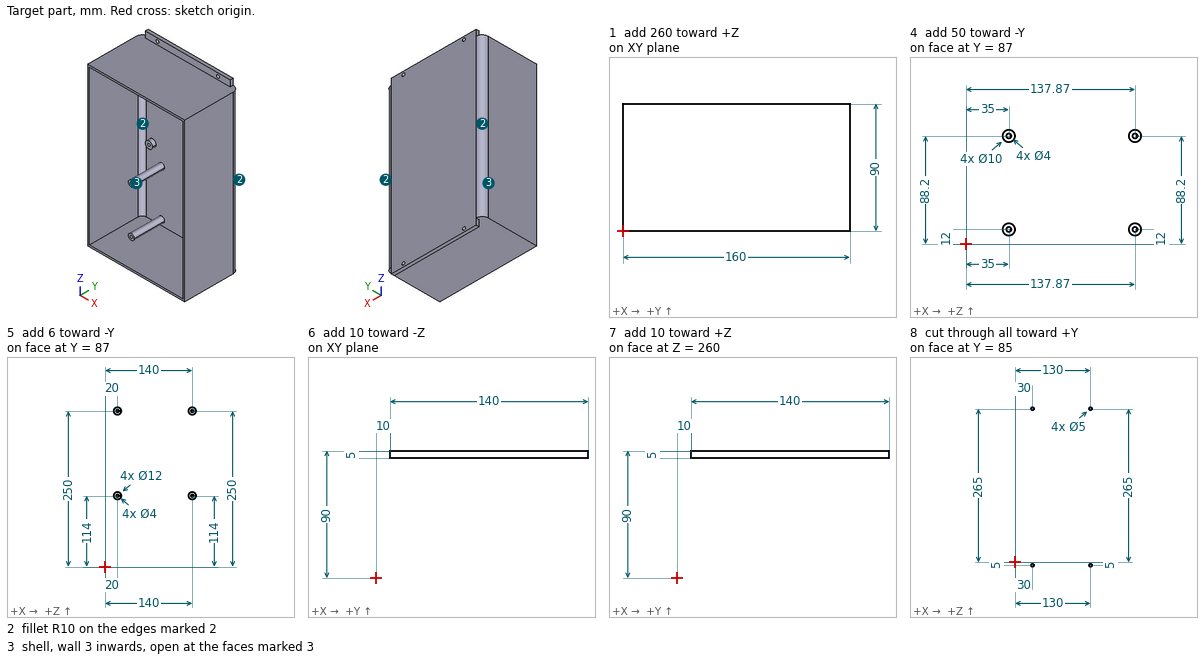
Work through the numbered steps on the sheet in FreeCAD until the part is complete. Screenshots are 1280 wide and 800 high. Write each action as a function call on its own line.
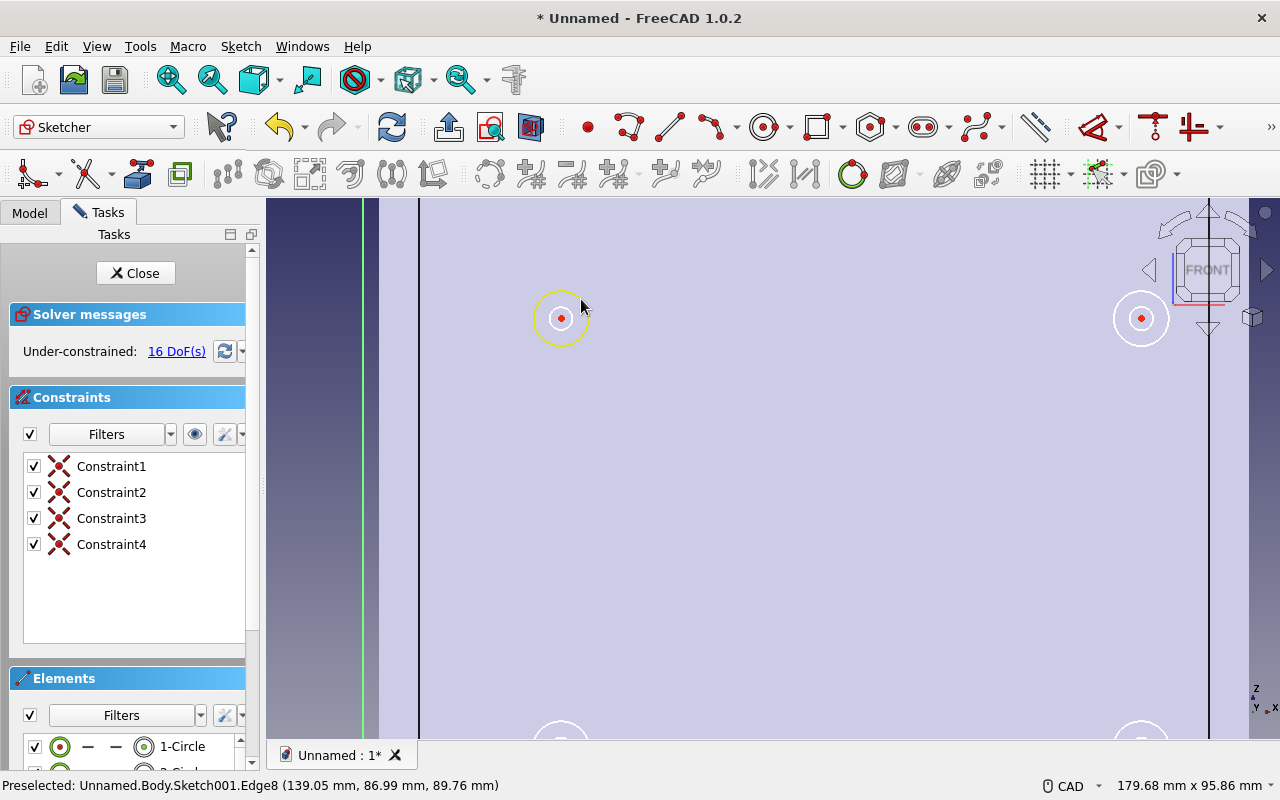
click(580, 299)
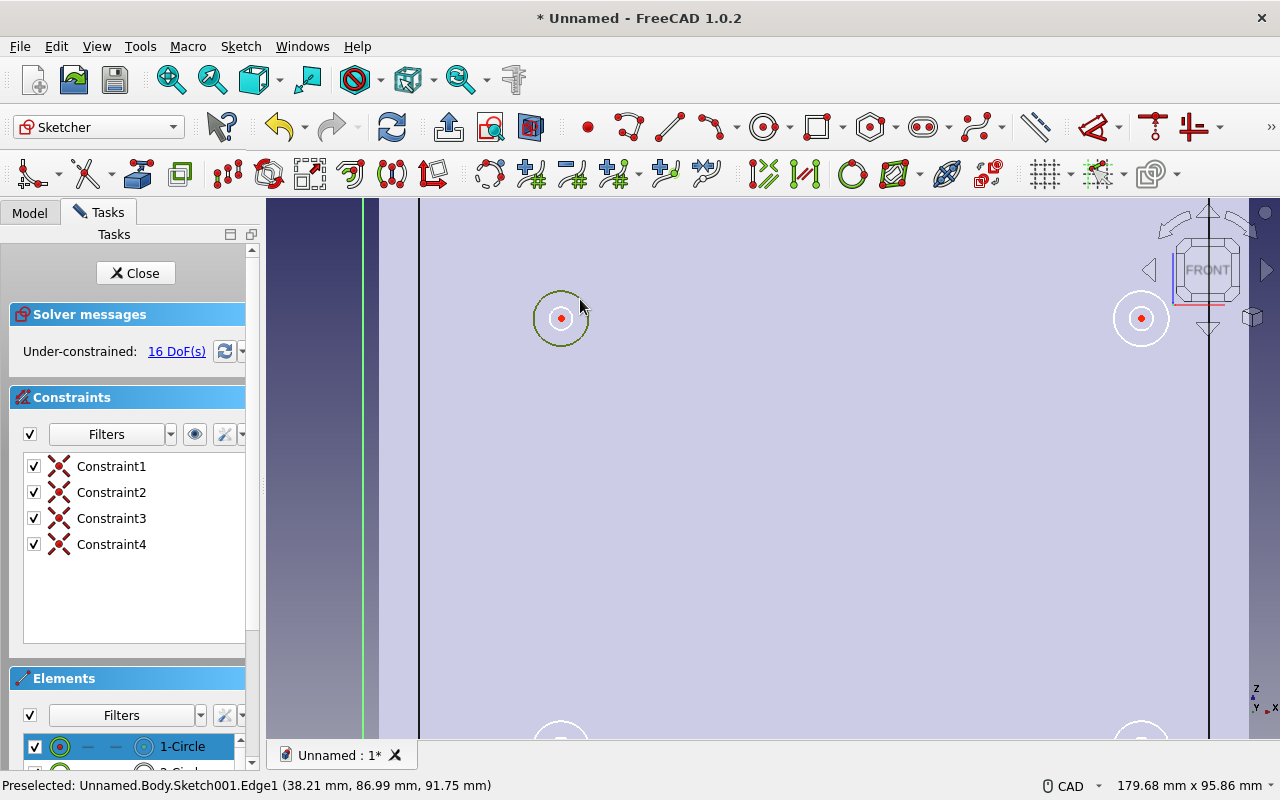
scroll(579, 298, down, 2)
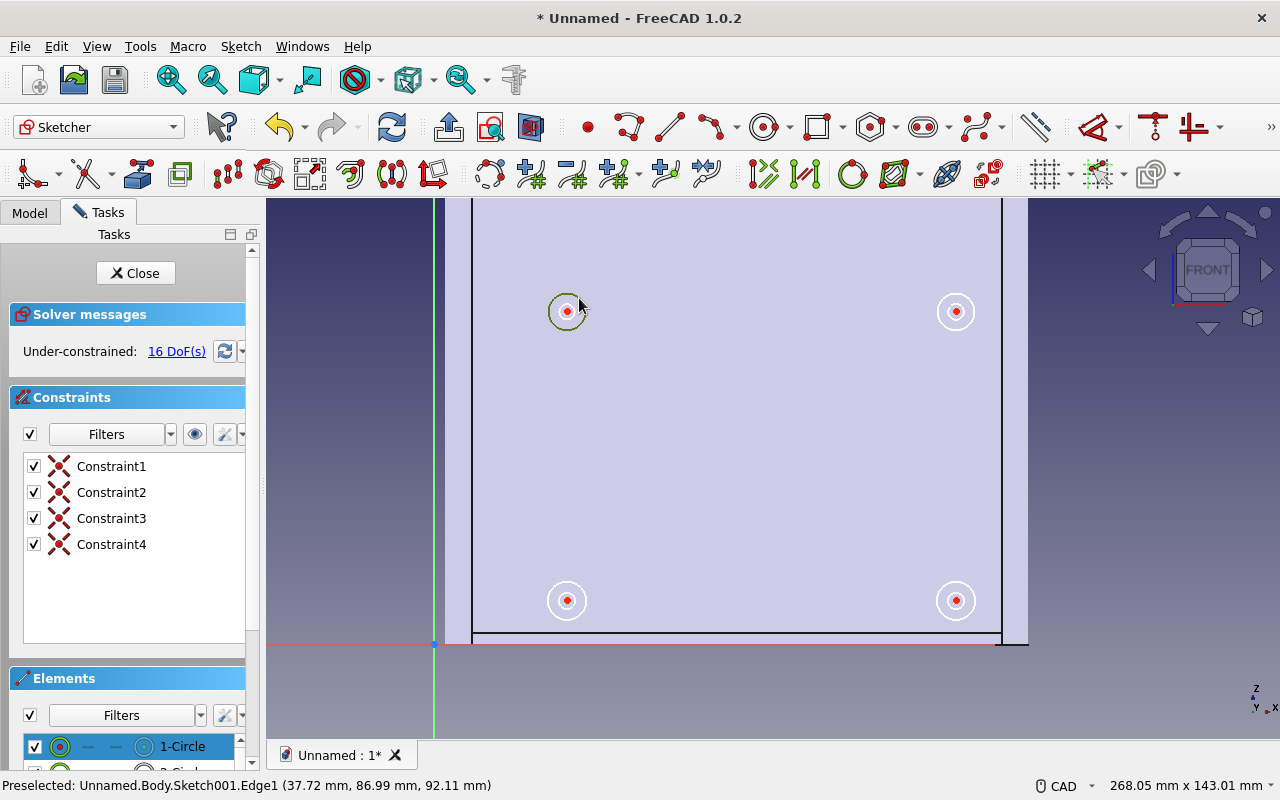
scroll(581, 587, up, 2)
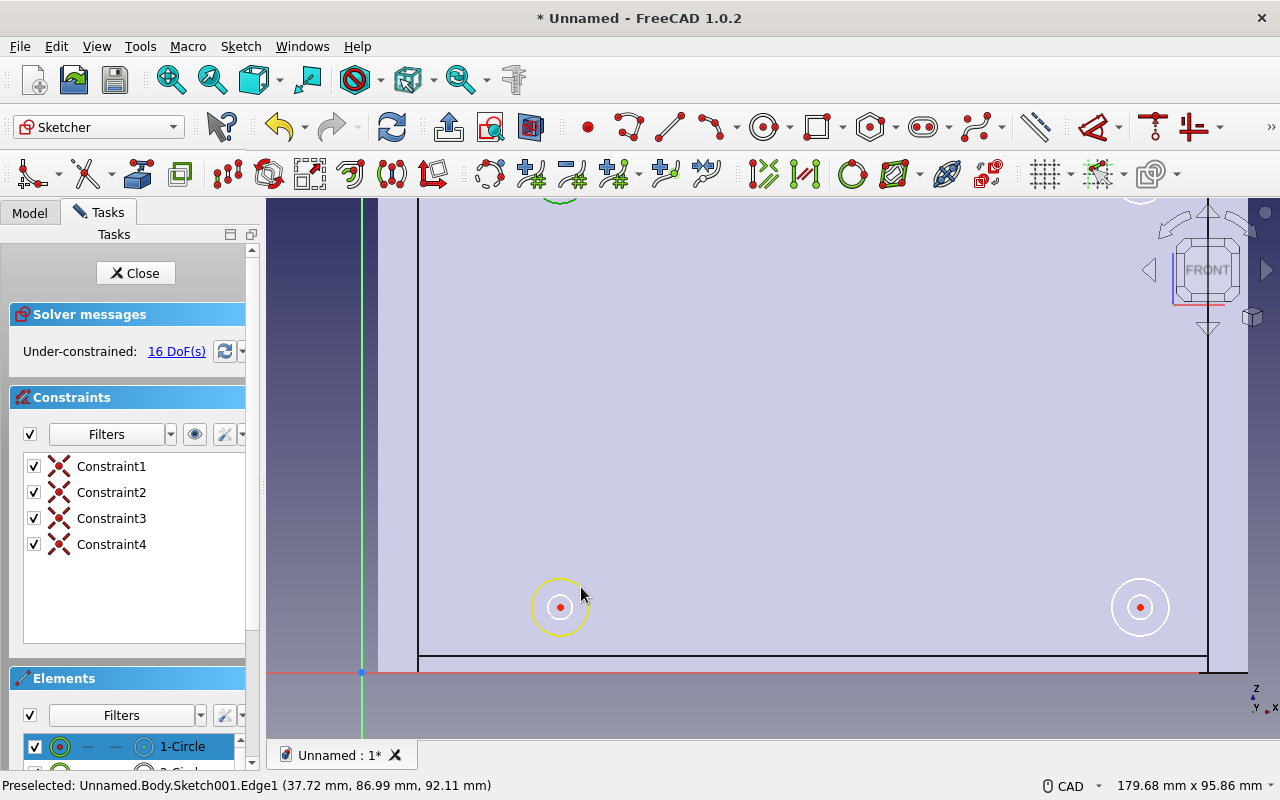
click(580, 587)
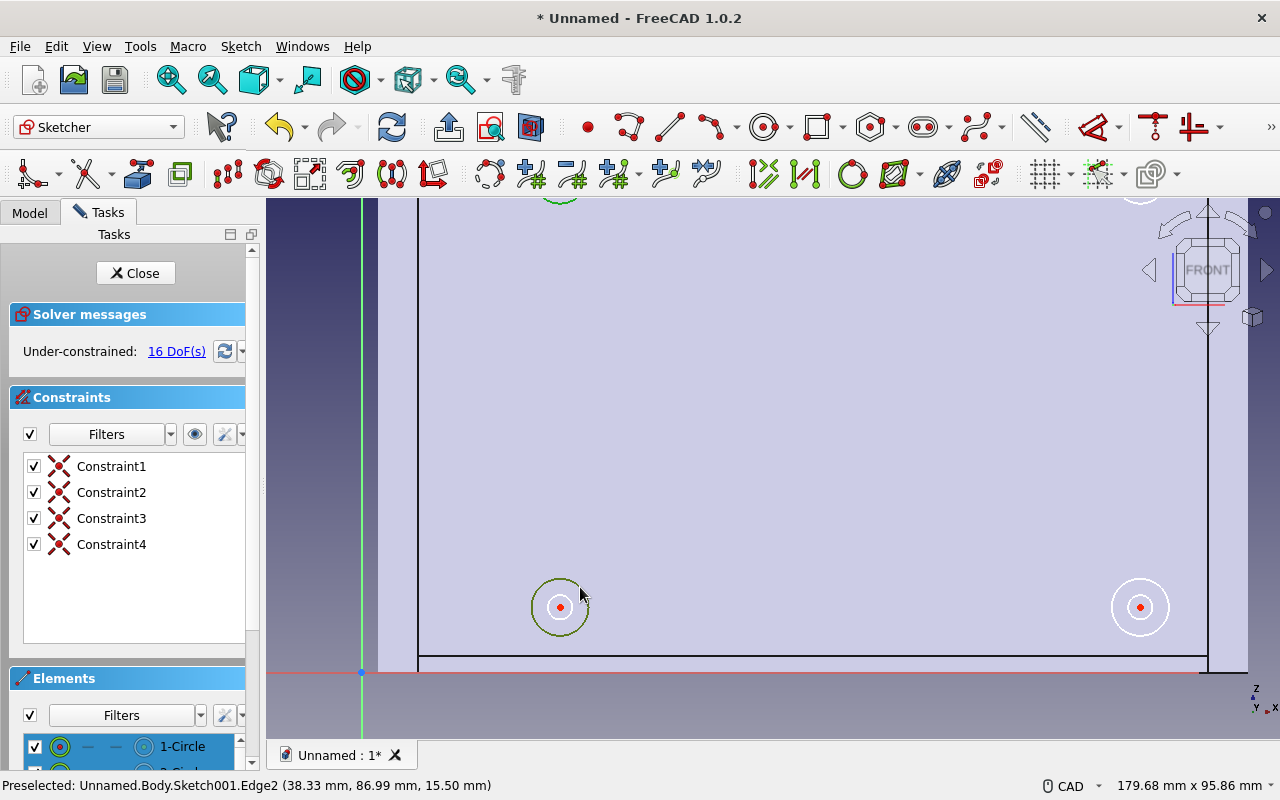
click(1112, 607)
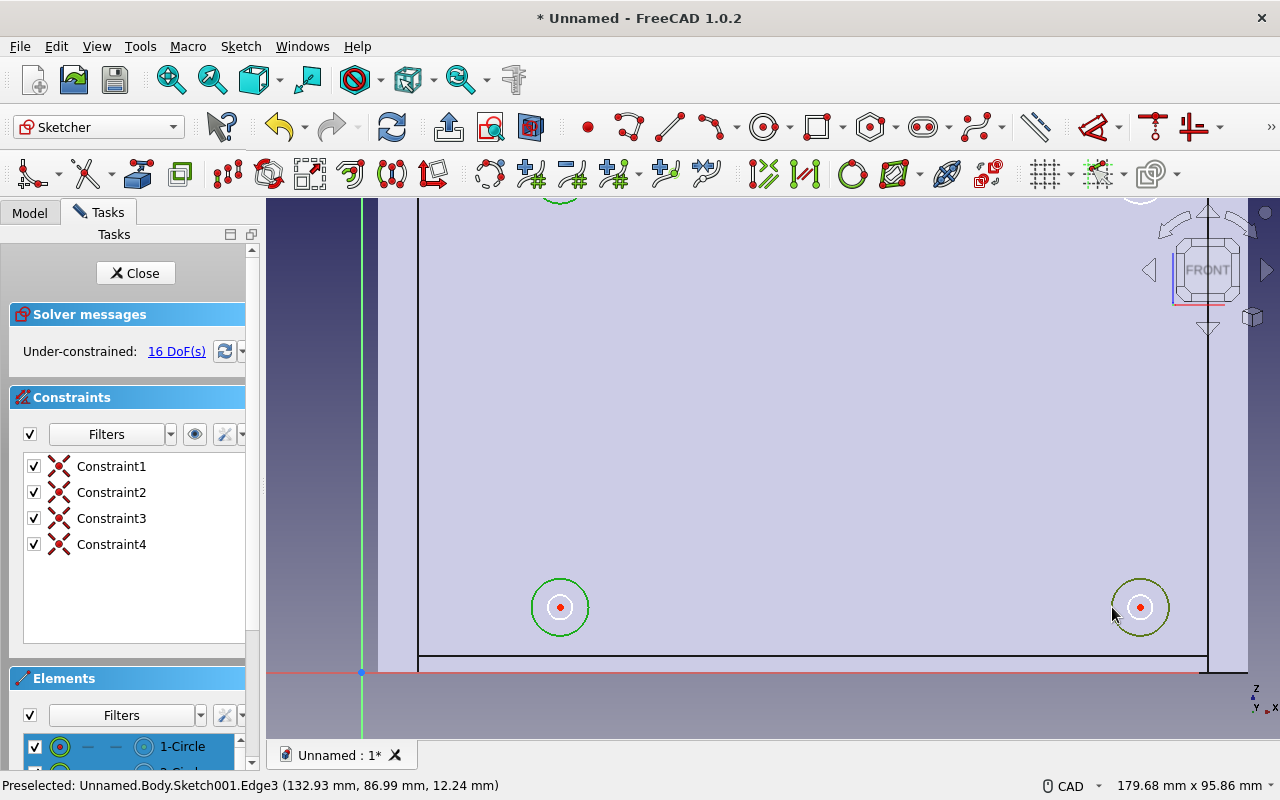
scroll(581, 588, down, 2)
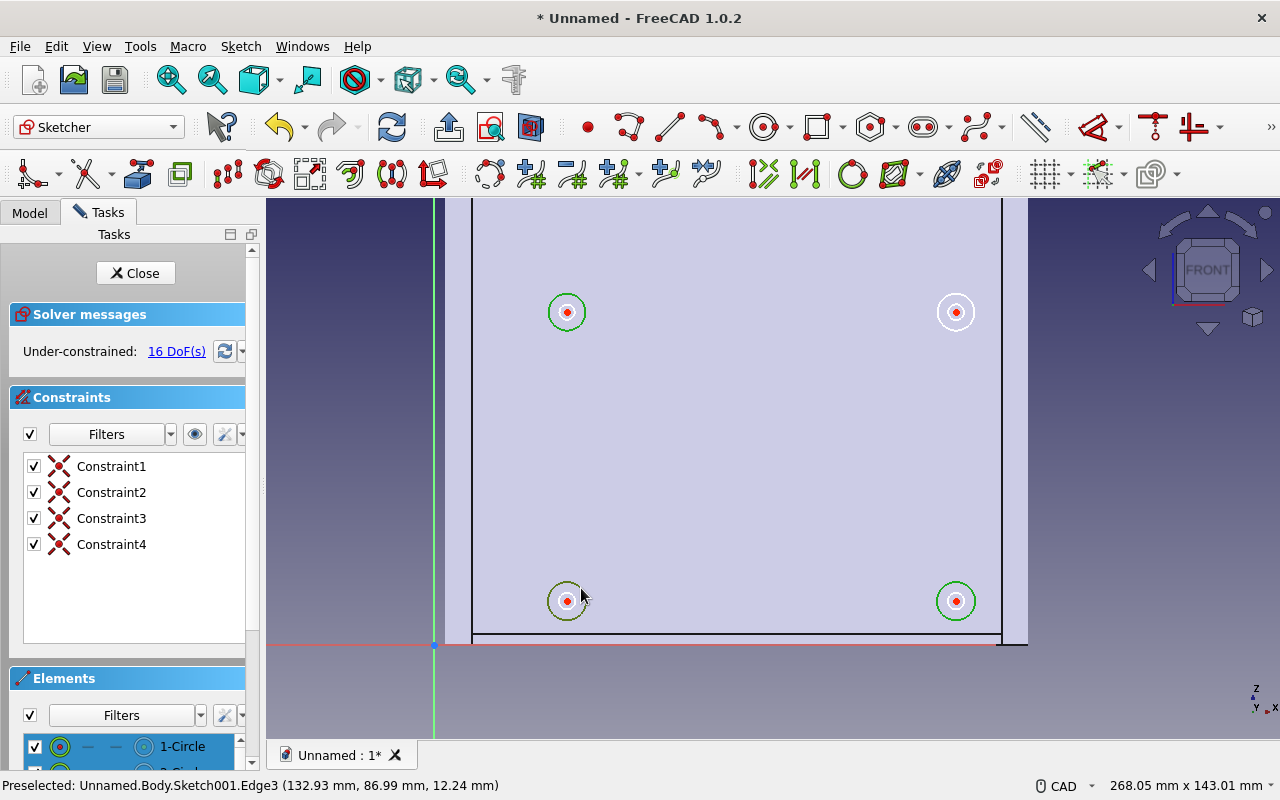
scroll(969, 299, up, 2)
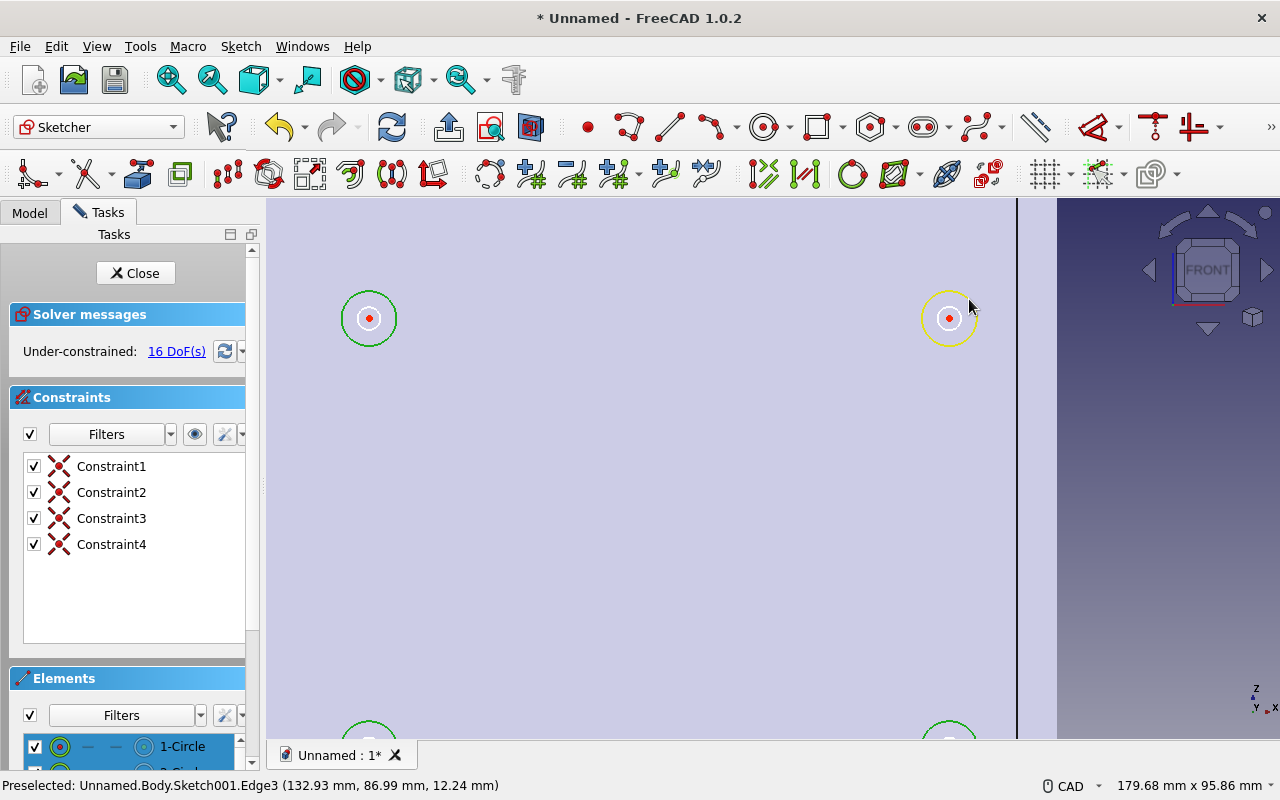
click(969, 299)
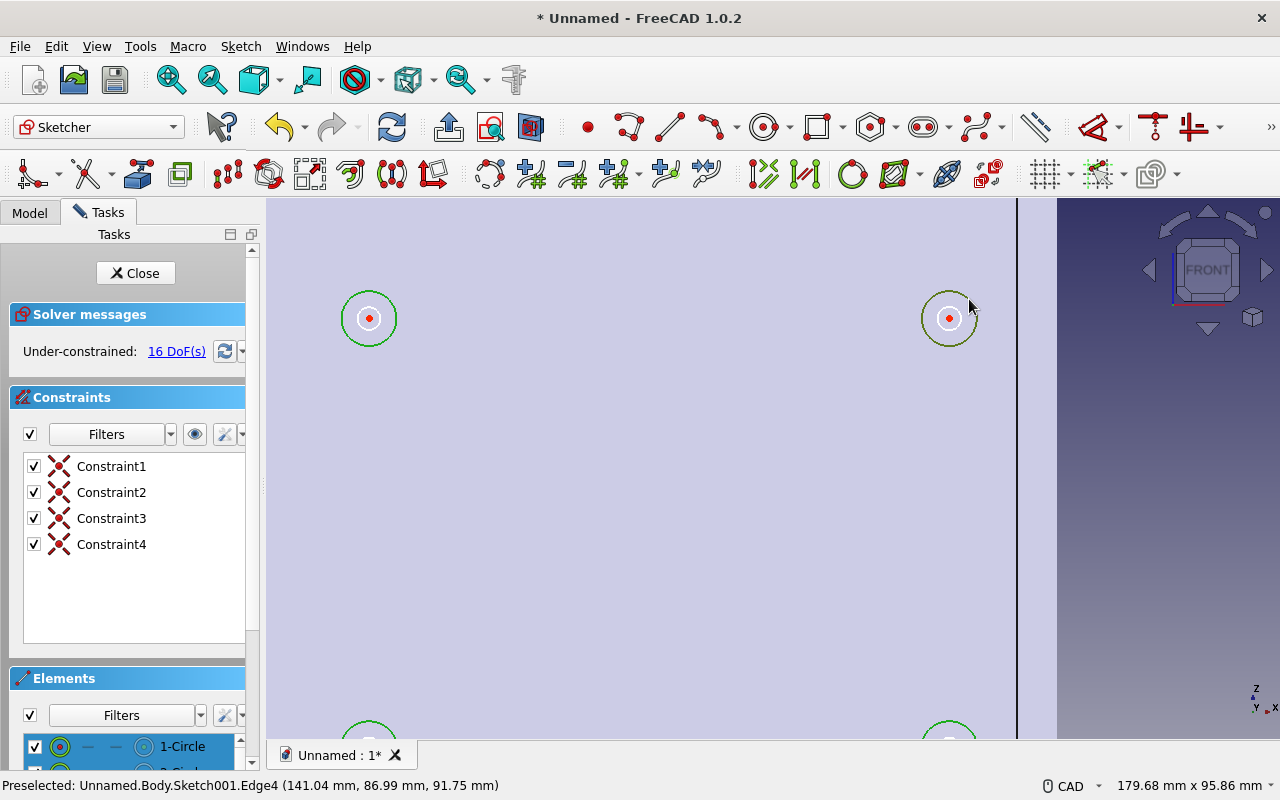
key(e)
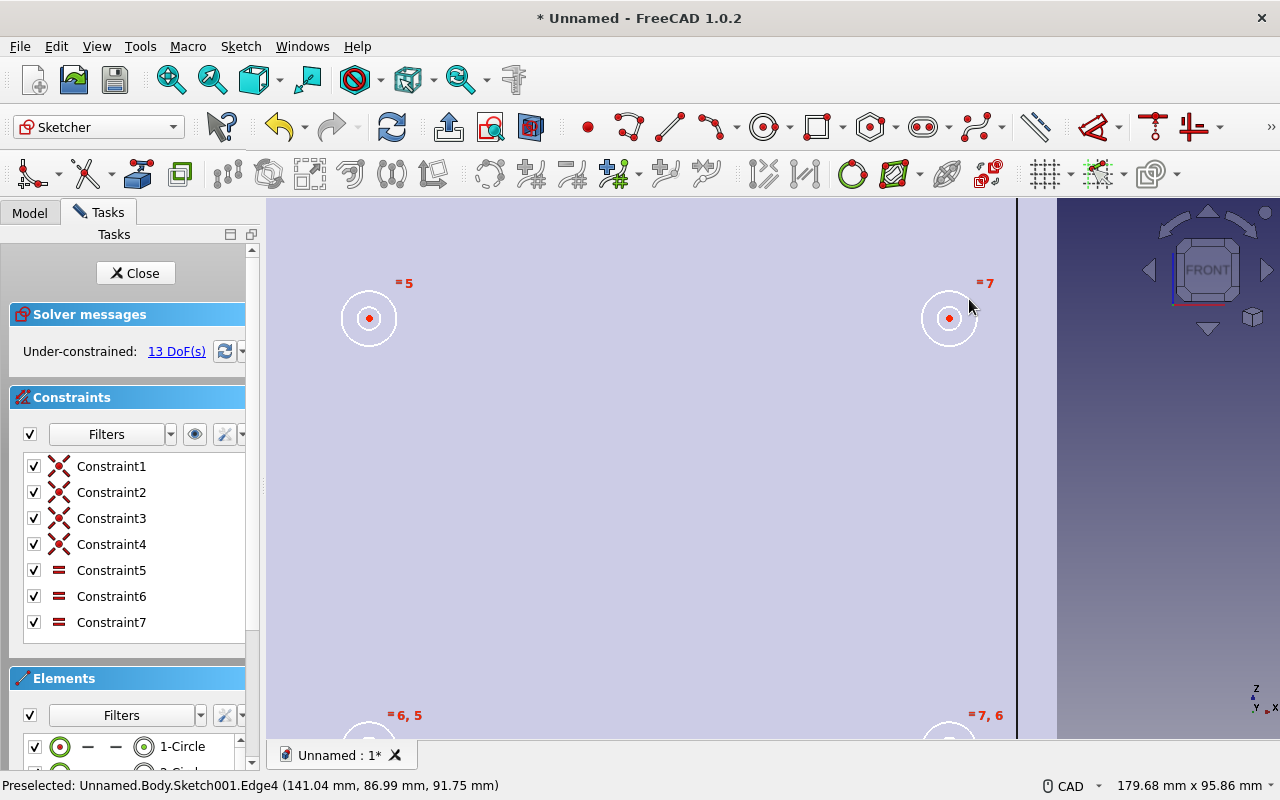
scroll(377, 311, up, 2)